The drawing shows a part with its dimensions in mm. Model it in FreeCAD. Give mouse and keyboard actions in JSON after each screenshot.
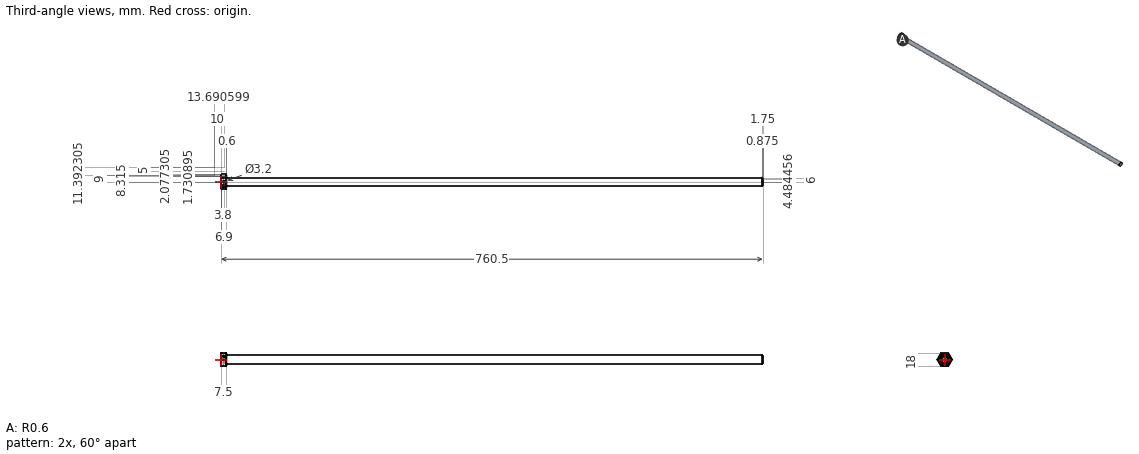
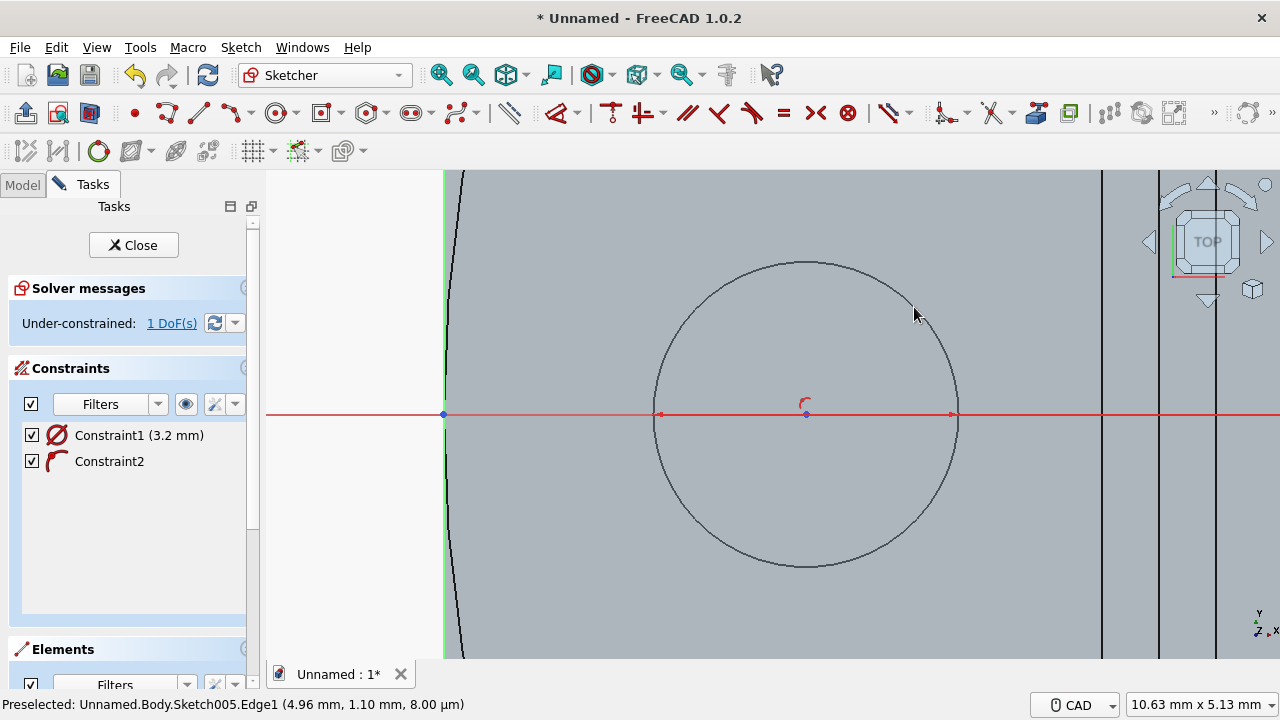
{"action": "key", "text": "d"}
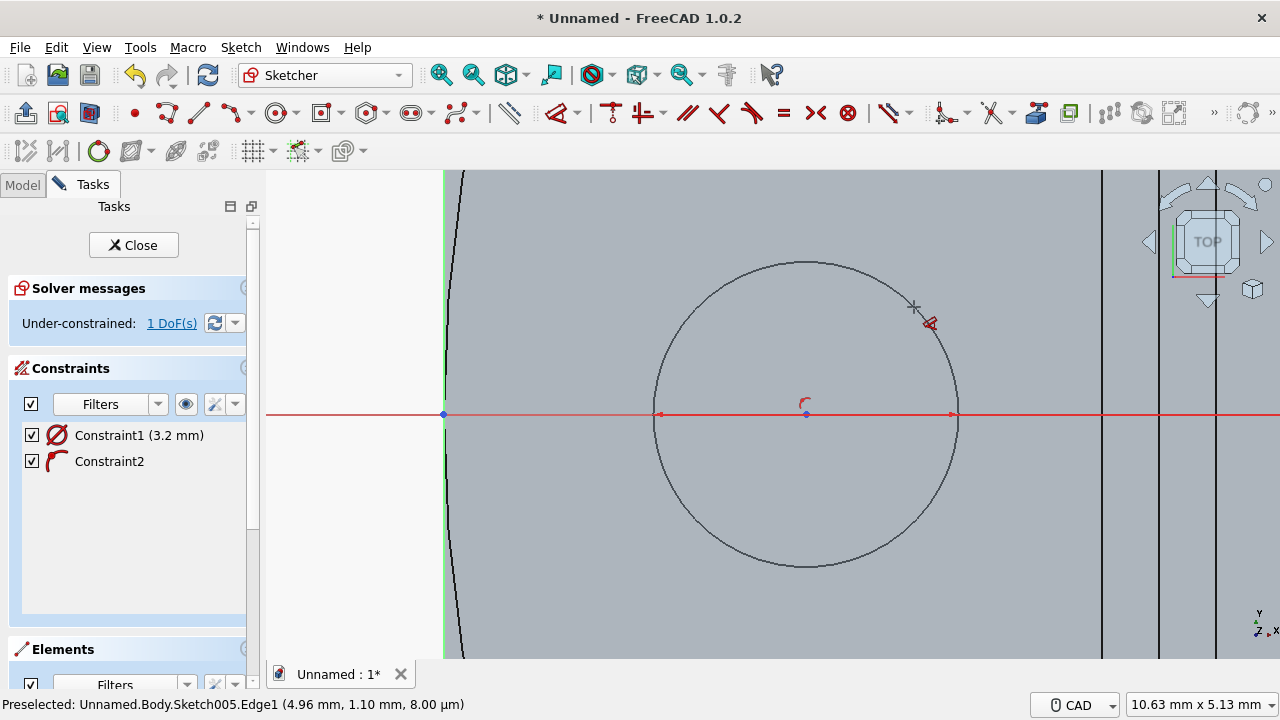
{"action": "left_click", "coordinate": [806, 414]}
{"action": "left_click", "coordinate": [625, 448]}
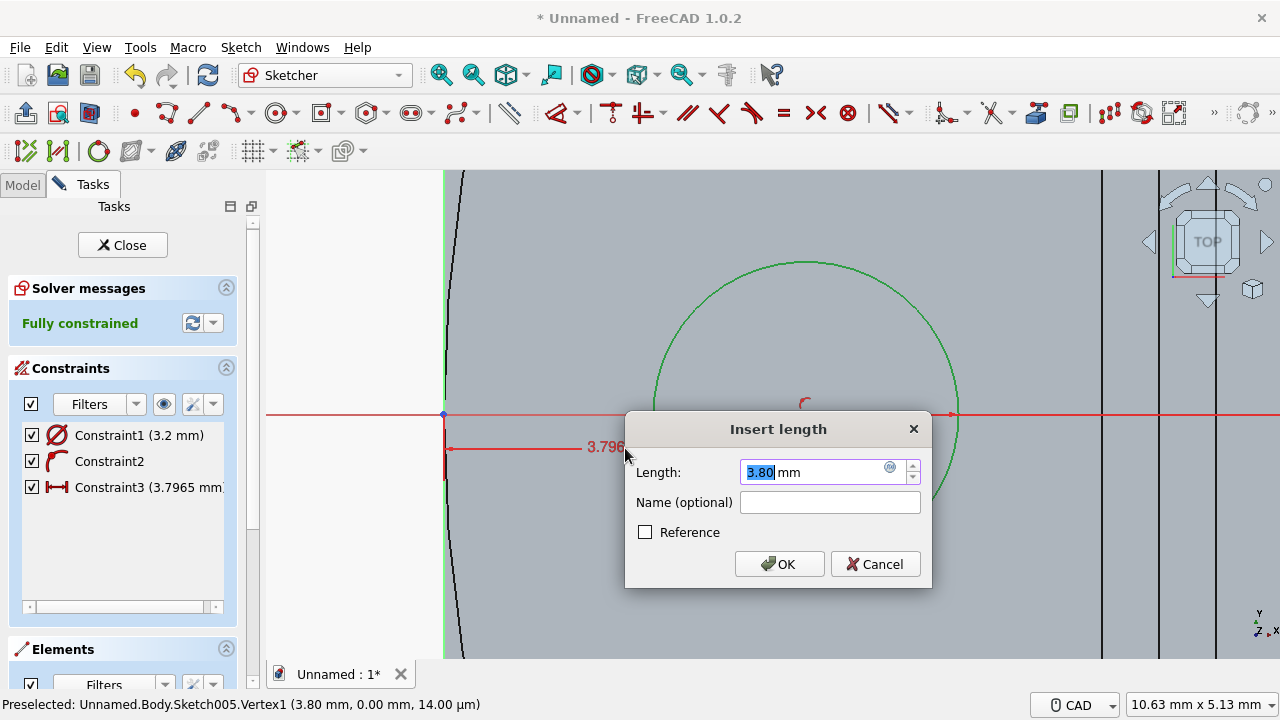
{"action": "type", "text": "3.8"}
{"action": "key", "text": "Return"}
{"action": "key", "text": "Escape"}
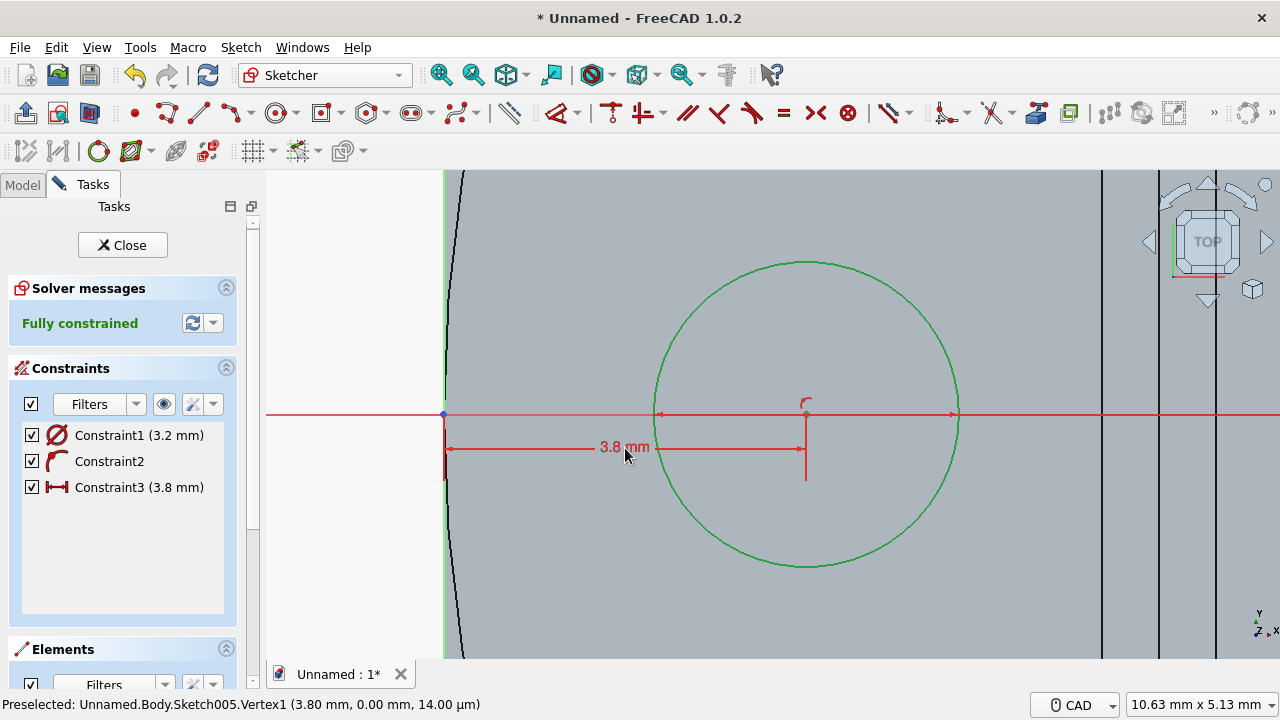
{"action": "left_click", "coordinate": [123, 245]}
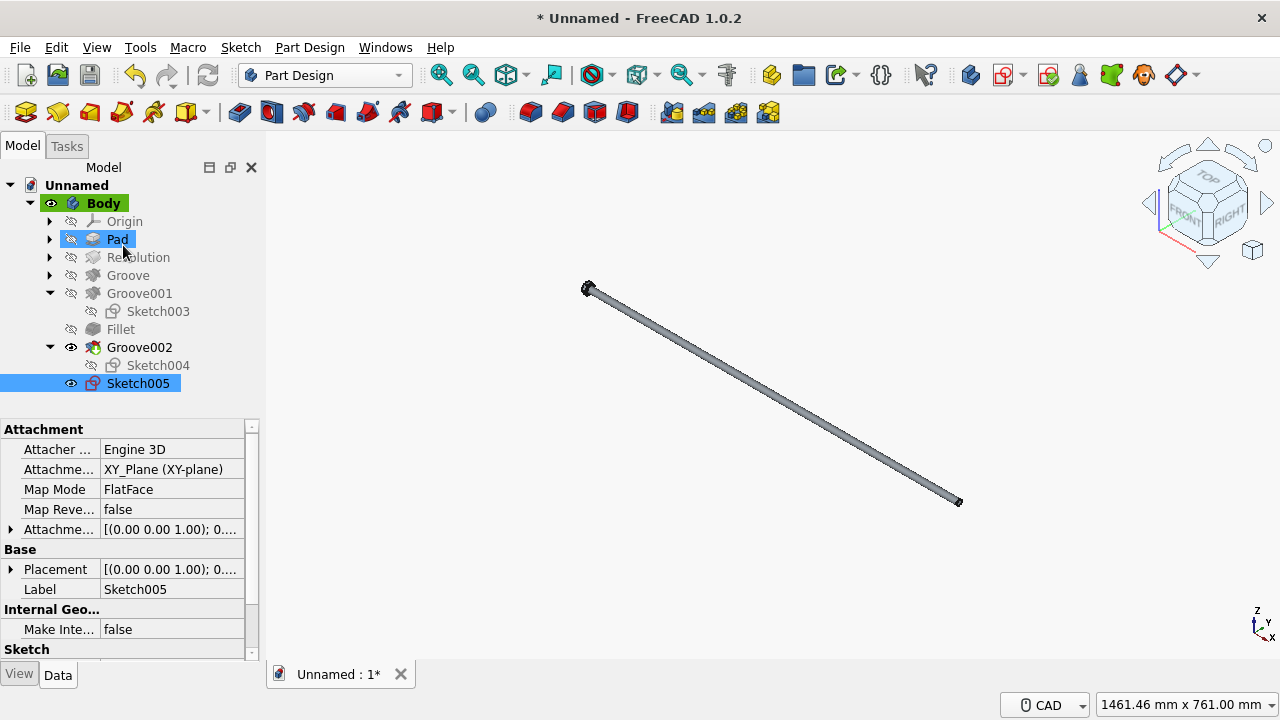
{"action": "left_click", "coordinate": [240, 112]}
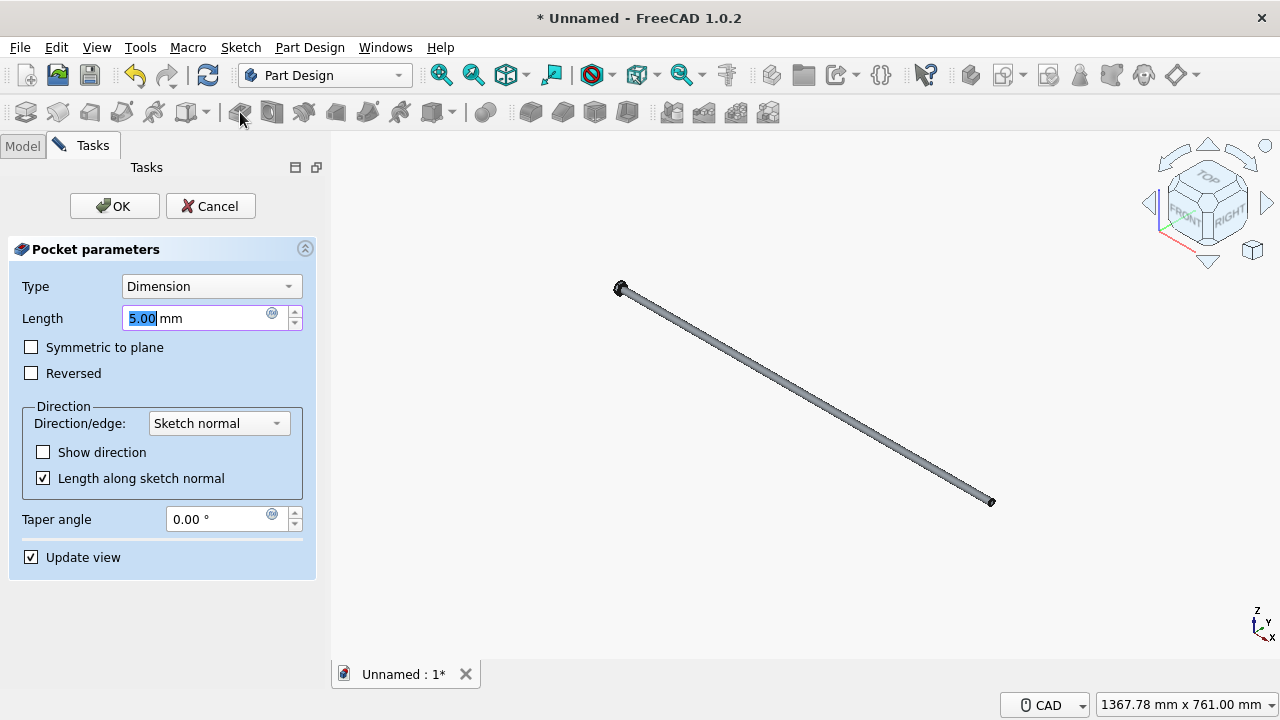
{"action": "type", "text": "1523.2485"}
{"action": "key", "text": "Tab"}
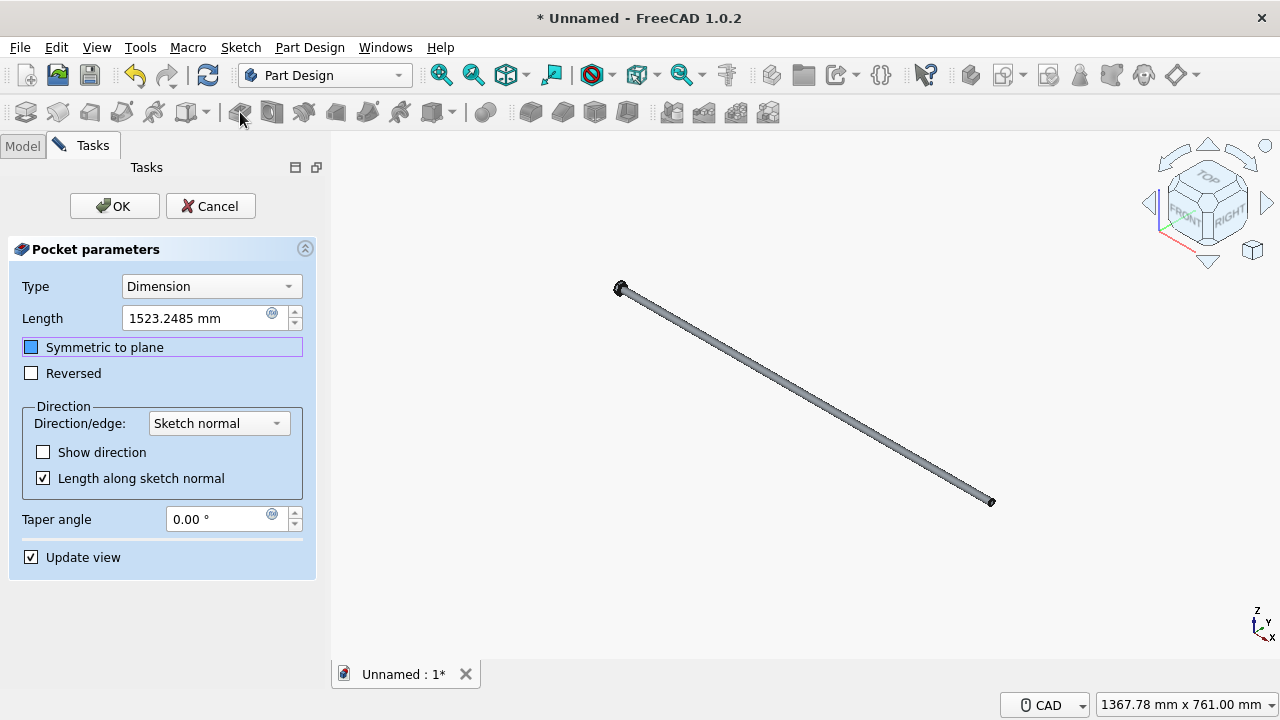
{"action": "left_click", "coordinate": [30, 347]}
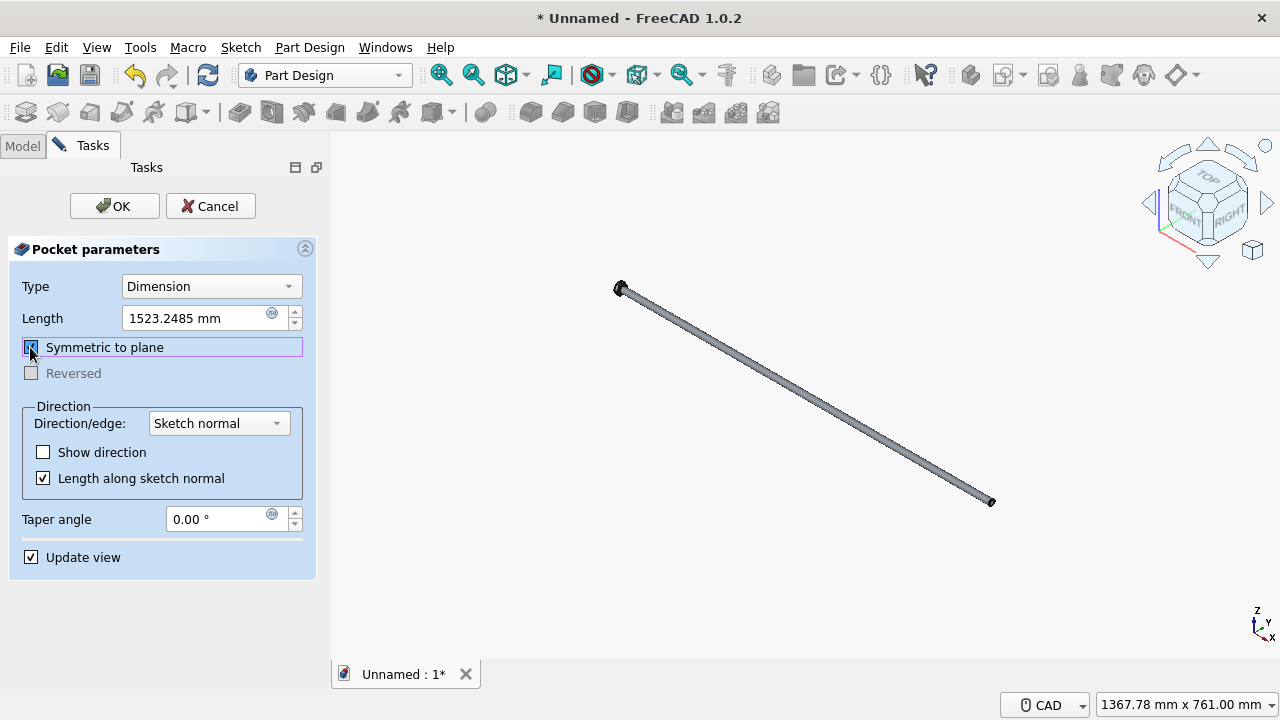
{"action": "left_click", "coordinate": [115, 206]}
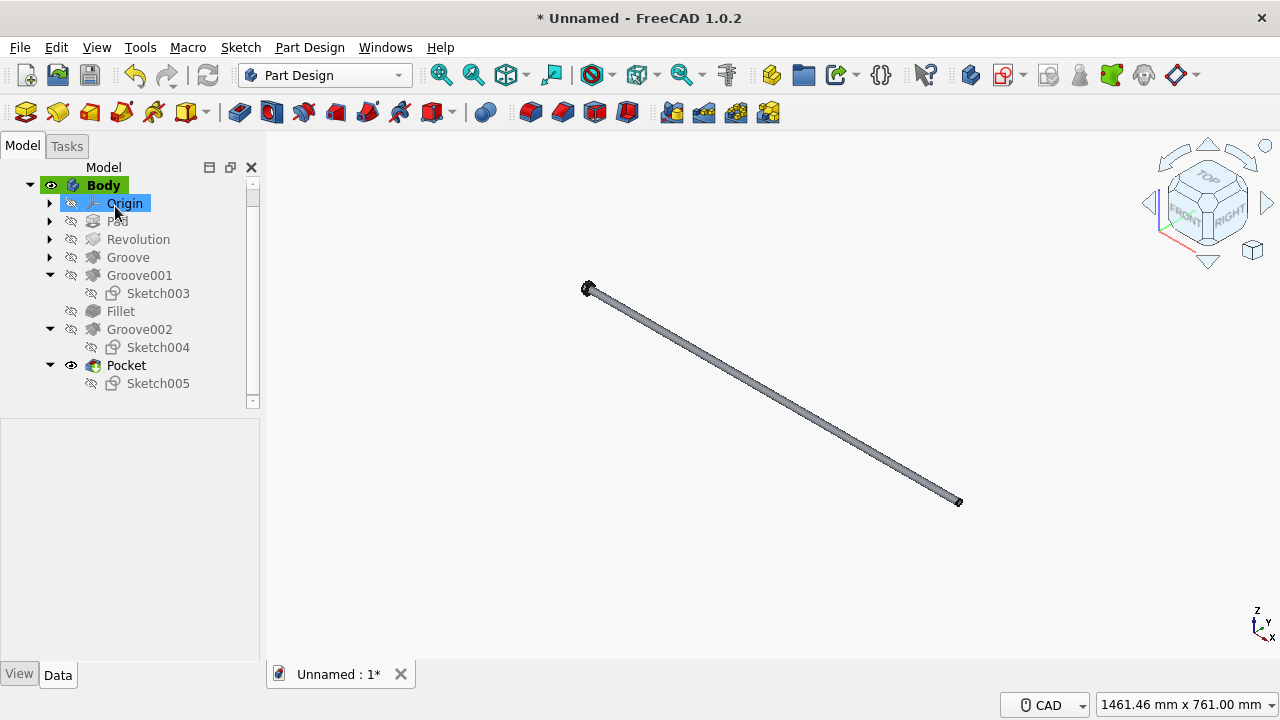
{"action": "key", "text": "v f"}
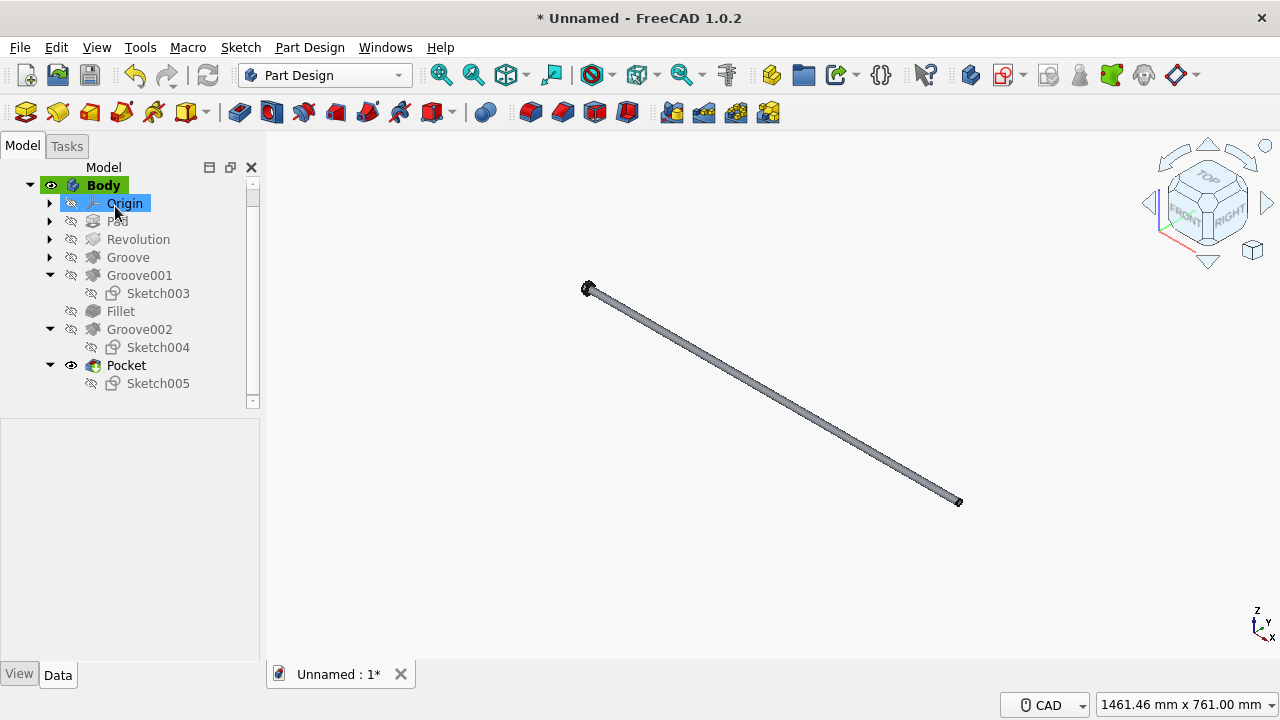
{"action": "left_click", "coordinate": [116, 365]}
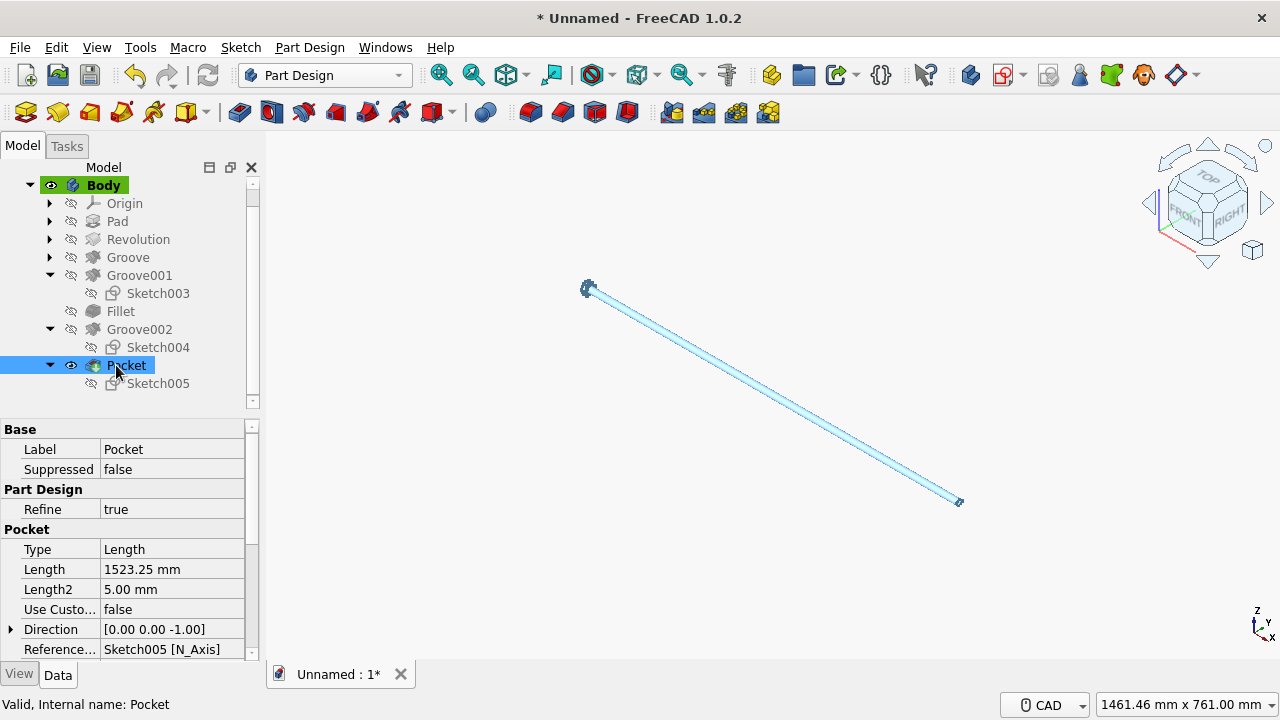
{"action": "left_click", "coordinate": [736, 112]}